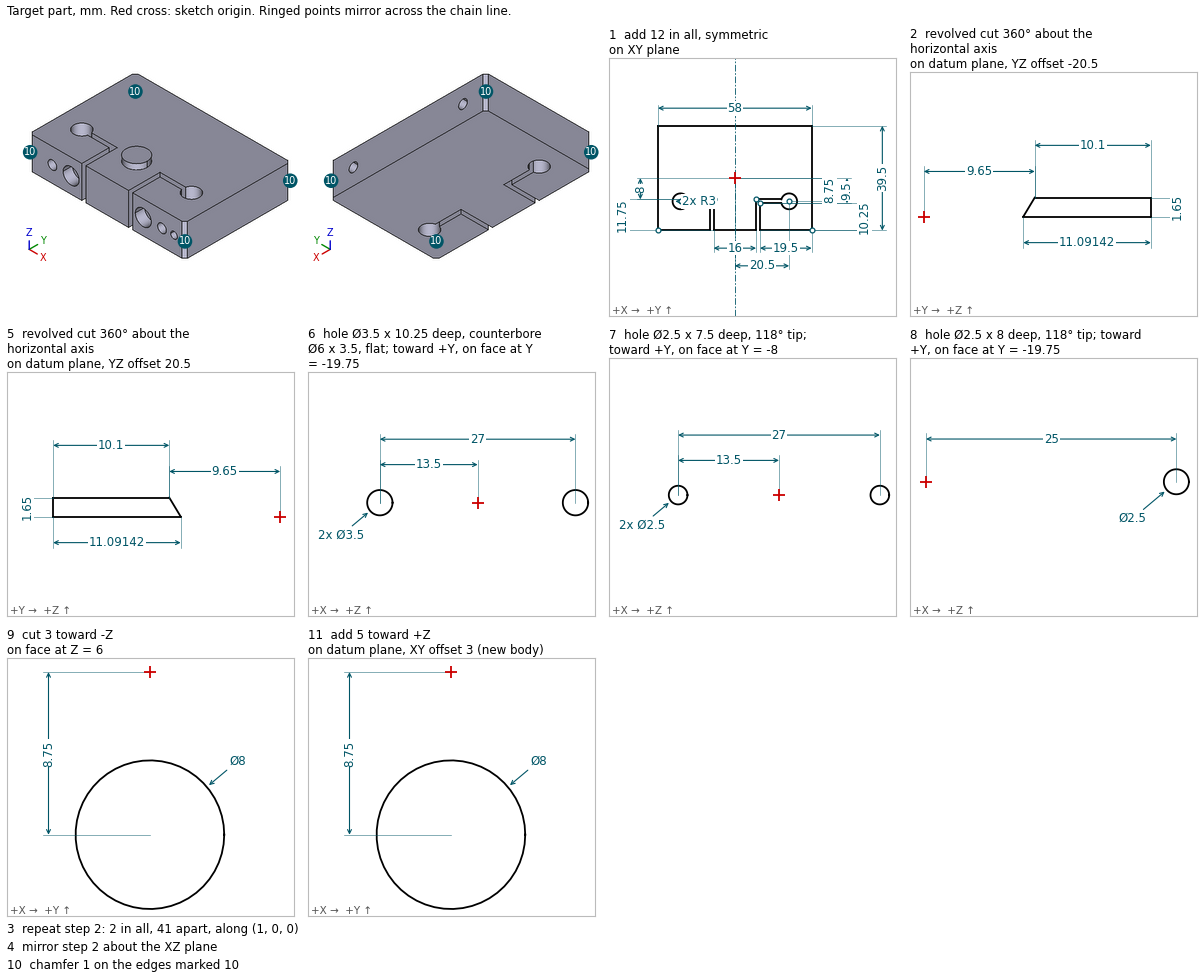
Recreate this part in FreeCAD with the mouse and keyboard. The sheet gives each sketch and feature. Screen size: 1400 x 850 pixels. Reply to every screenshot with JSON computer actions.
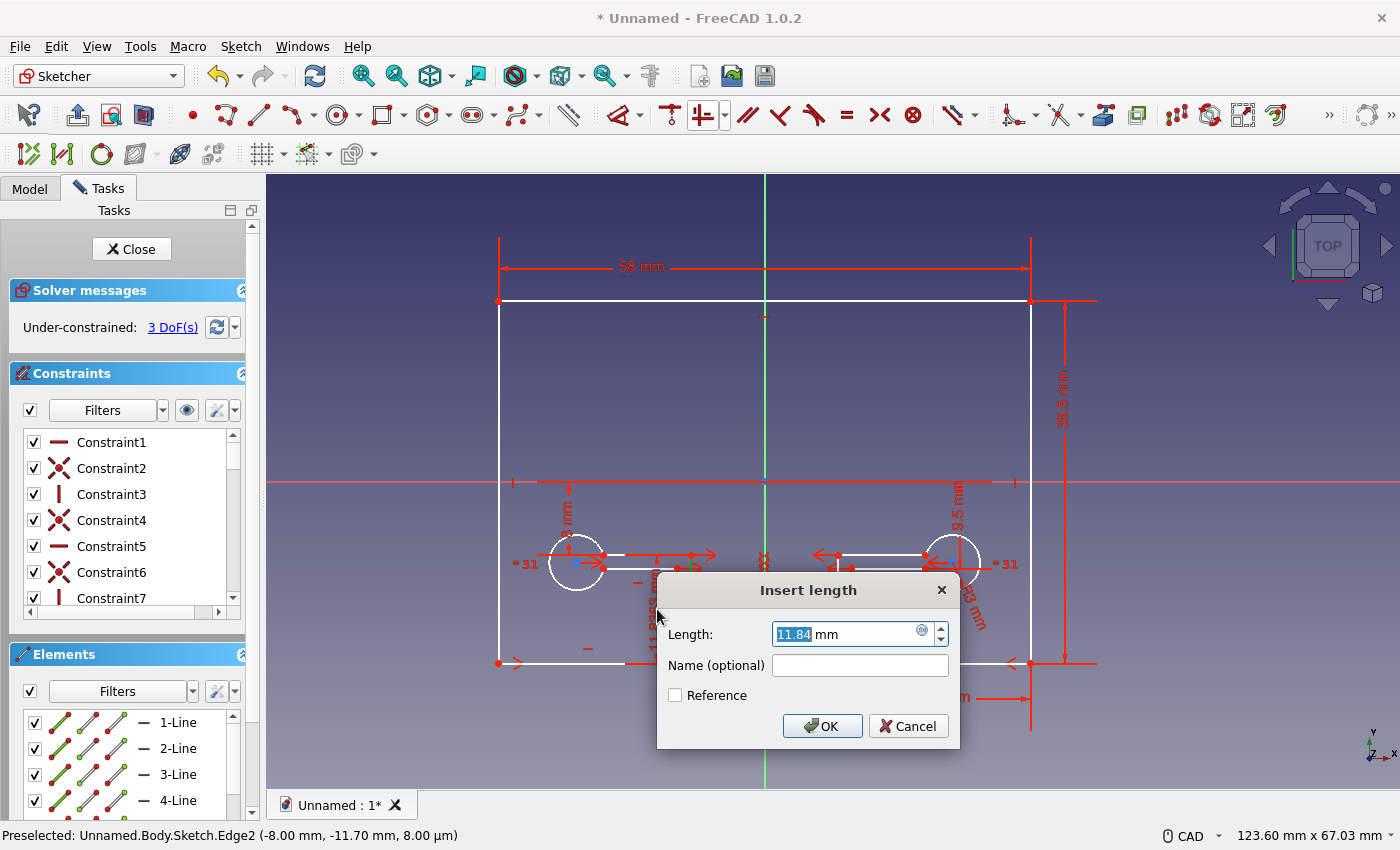
{"action": "type", "text": "11.75"}
{"action": "key", "text": "Return"}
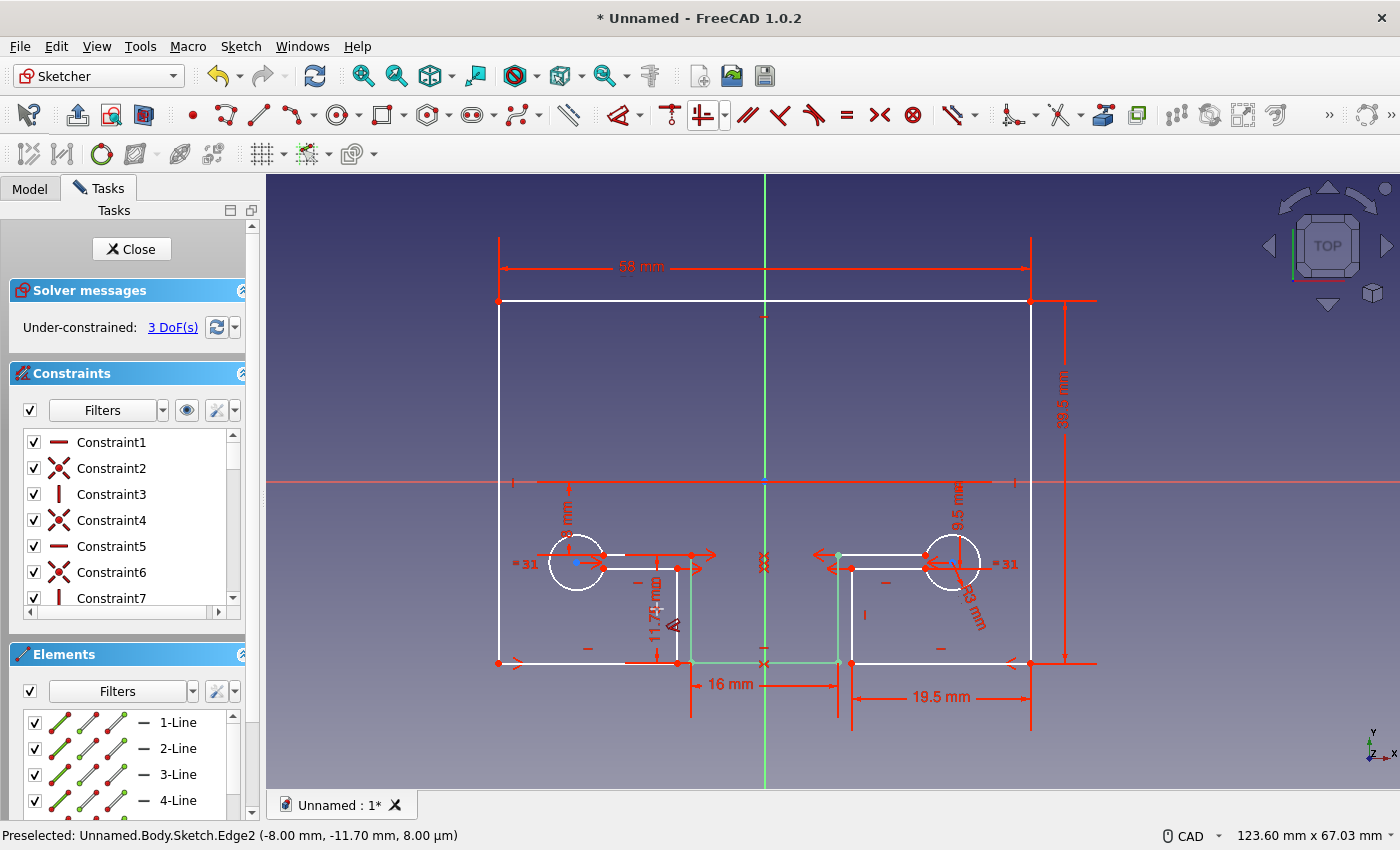
{"action": "left_click", "coordinate": [852, 597]}
{"action": "left_click", "coordinate": [886, 616]}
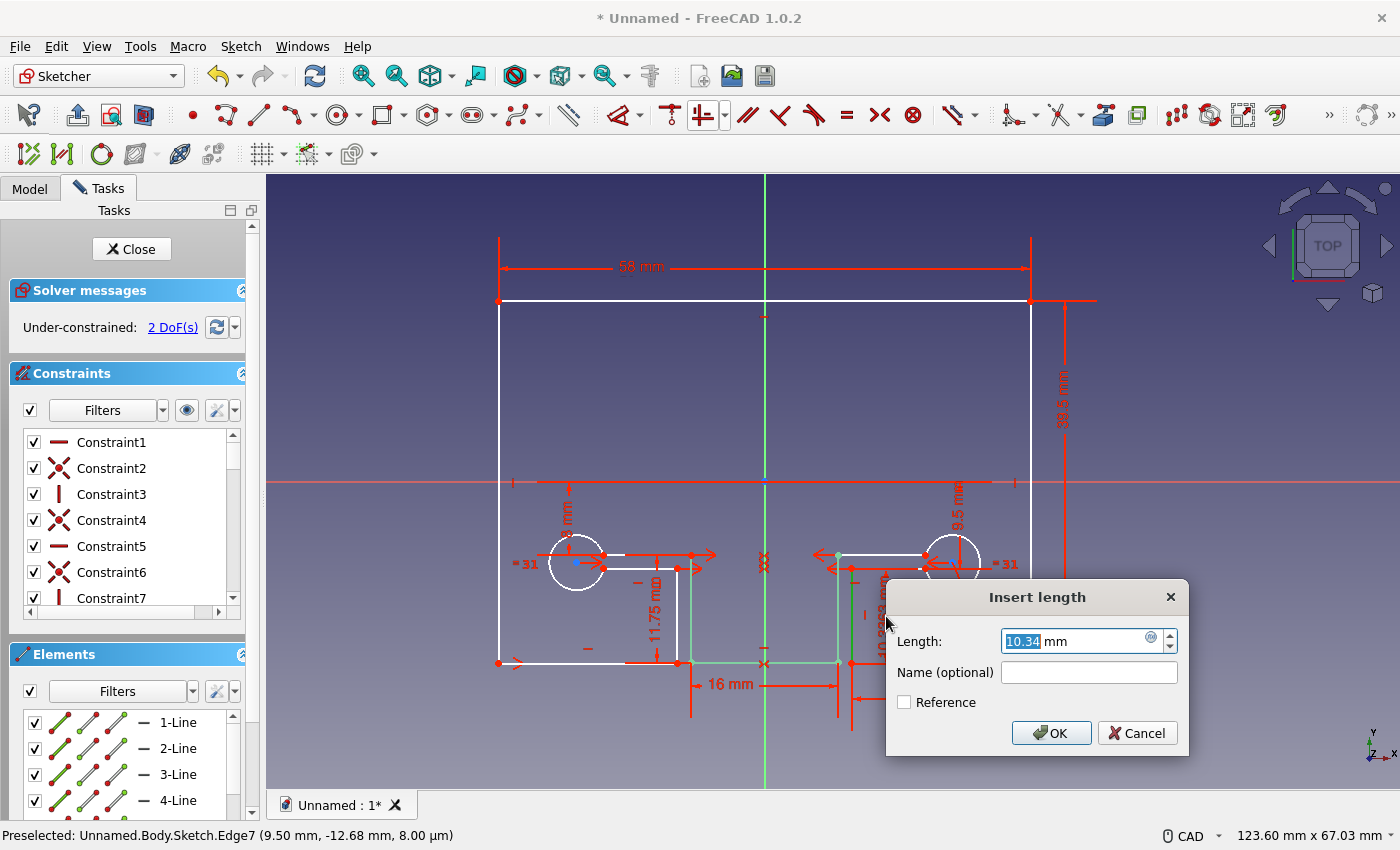
{"action": "type", "text": "10.25"}
{"action": "key", "text": "Return"}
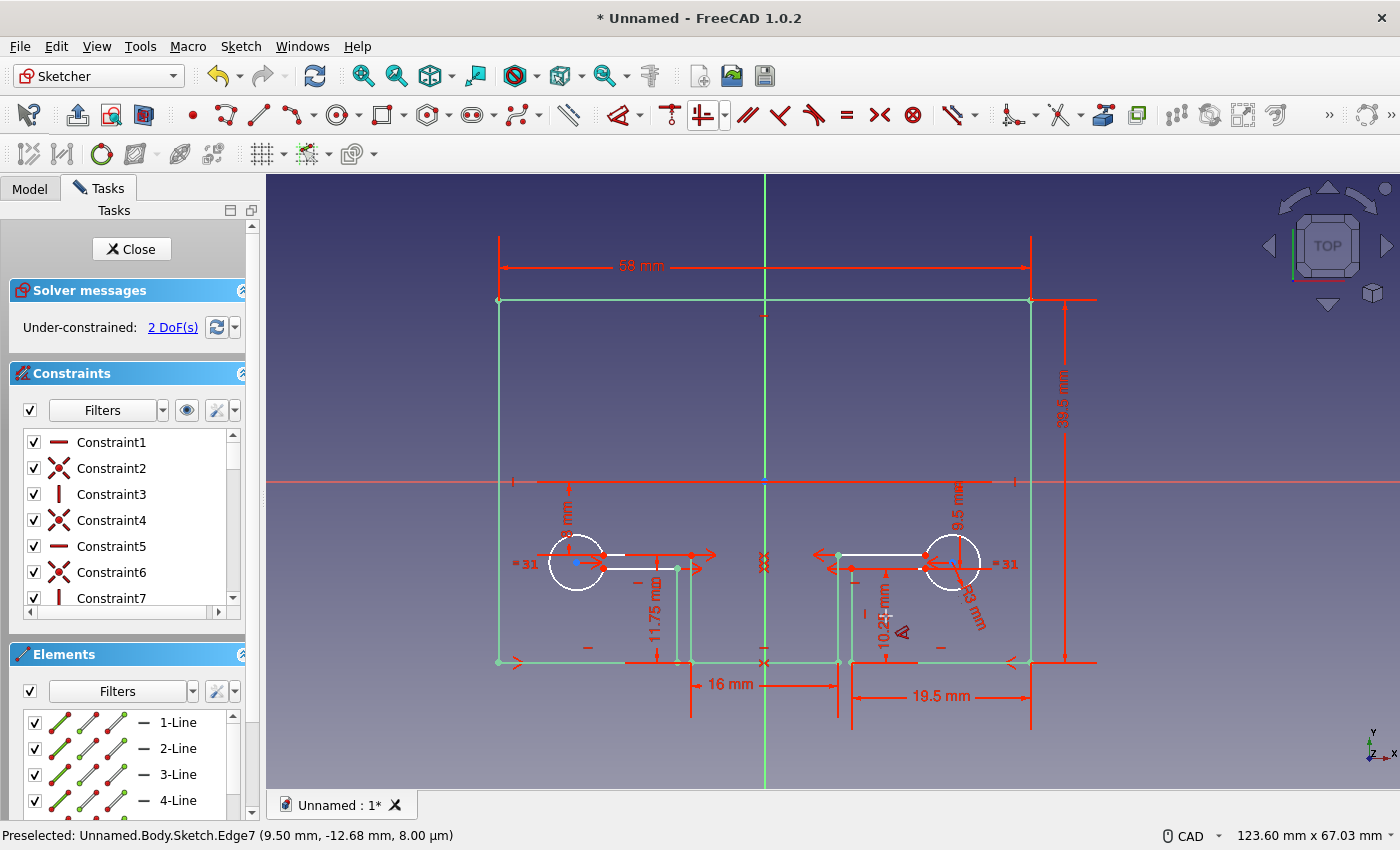
{"action": "left_click", "coordinate": [952, 563]}
{"action": "left_click", "coordinate": [815, 597]}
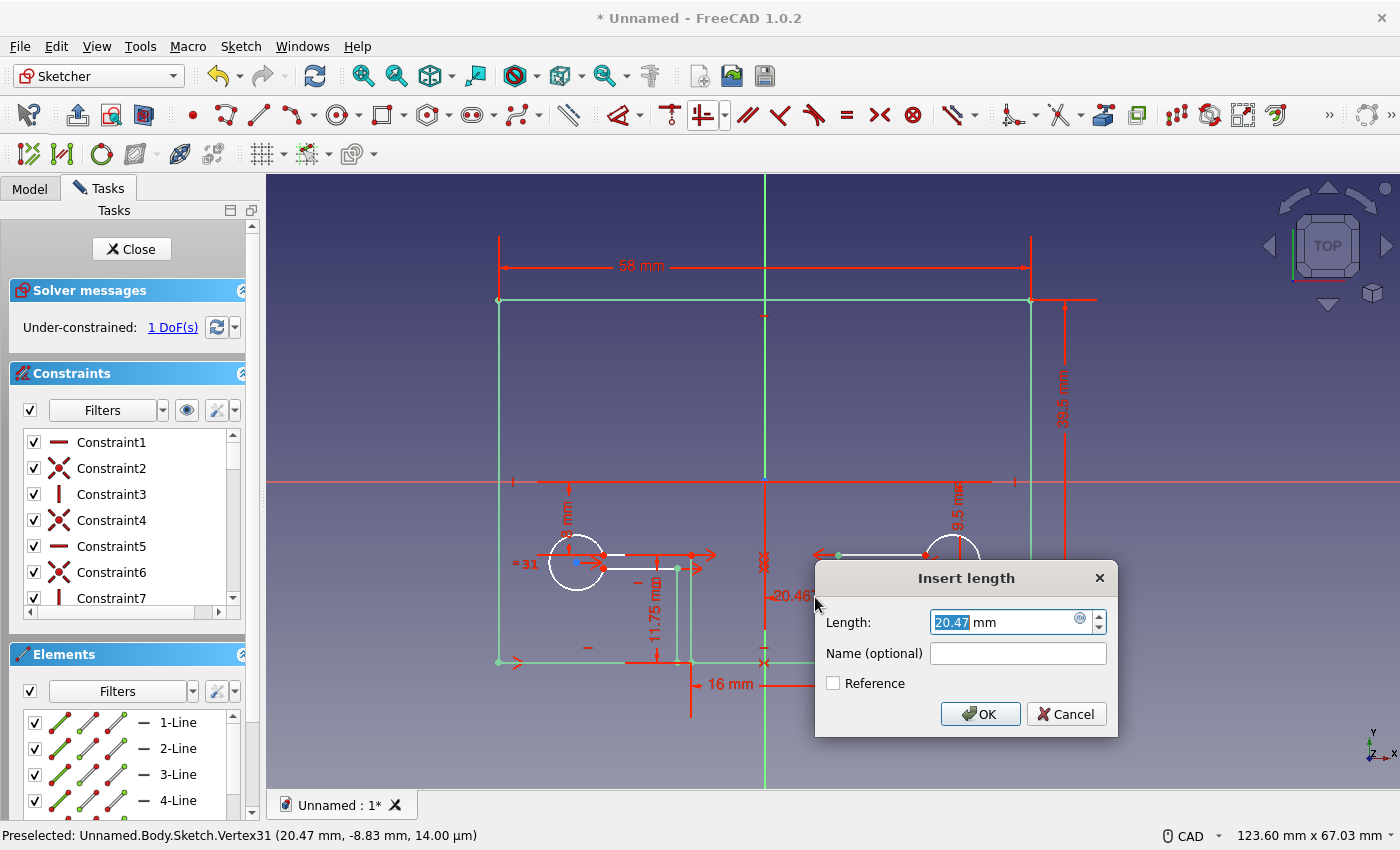
{"action": "type", "text": "20.5"}
{"action": "key", "text": "Return"}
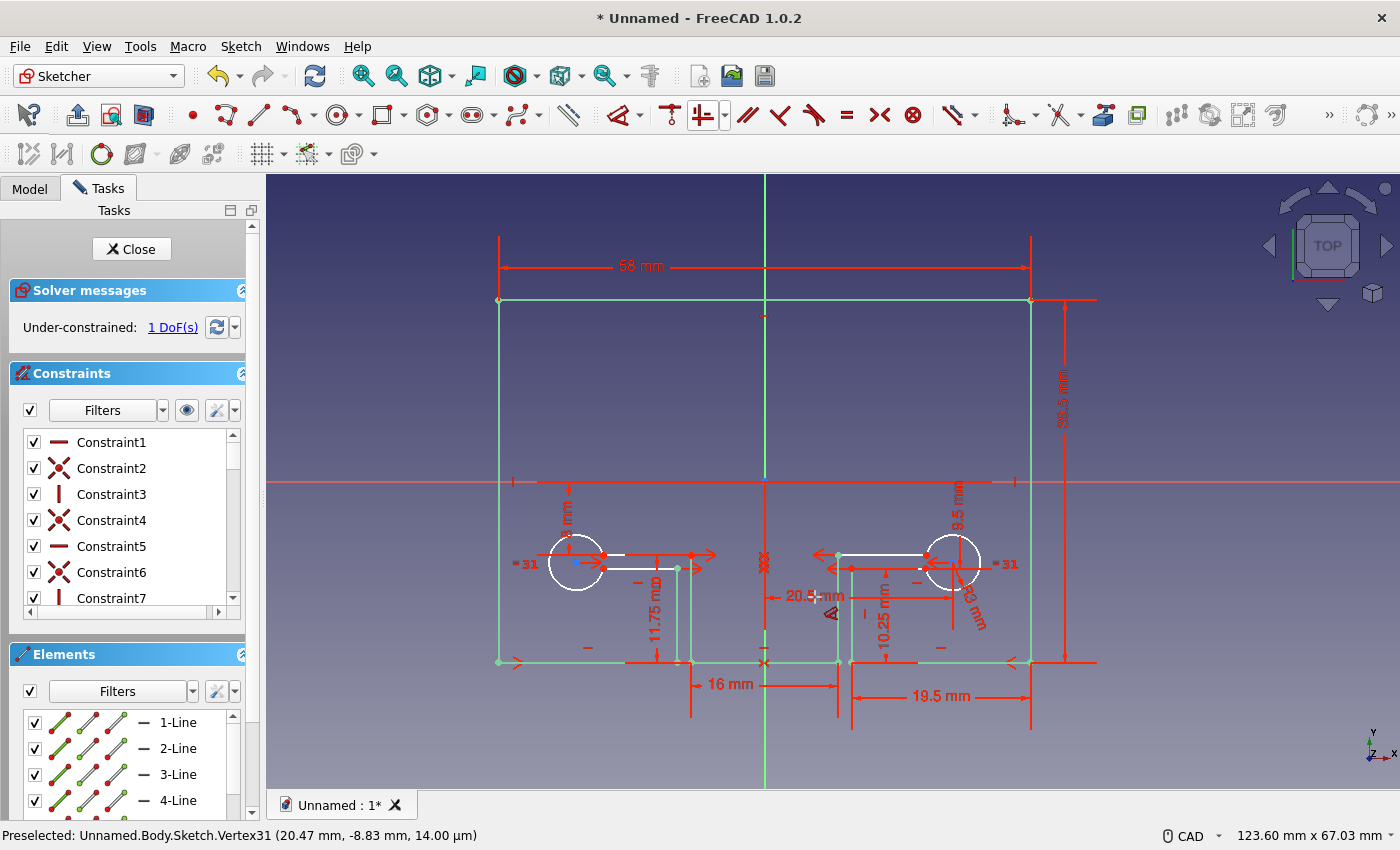
{"action": "left_click", "coordinate": [953, 563]}
{"action": "left_click", "coordinate": [731, 522]}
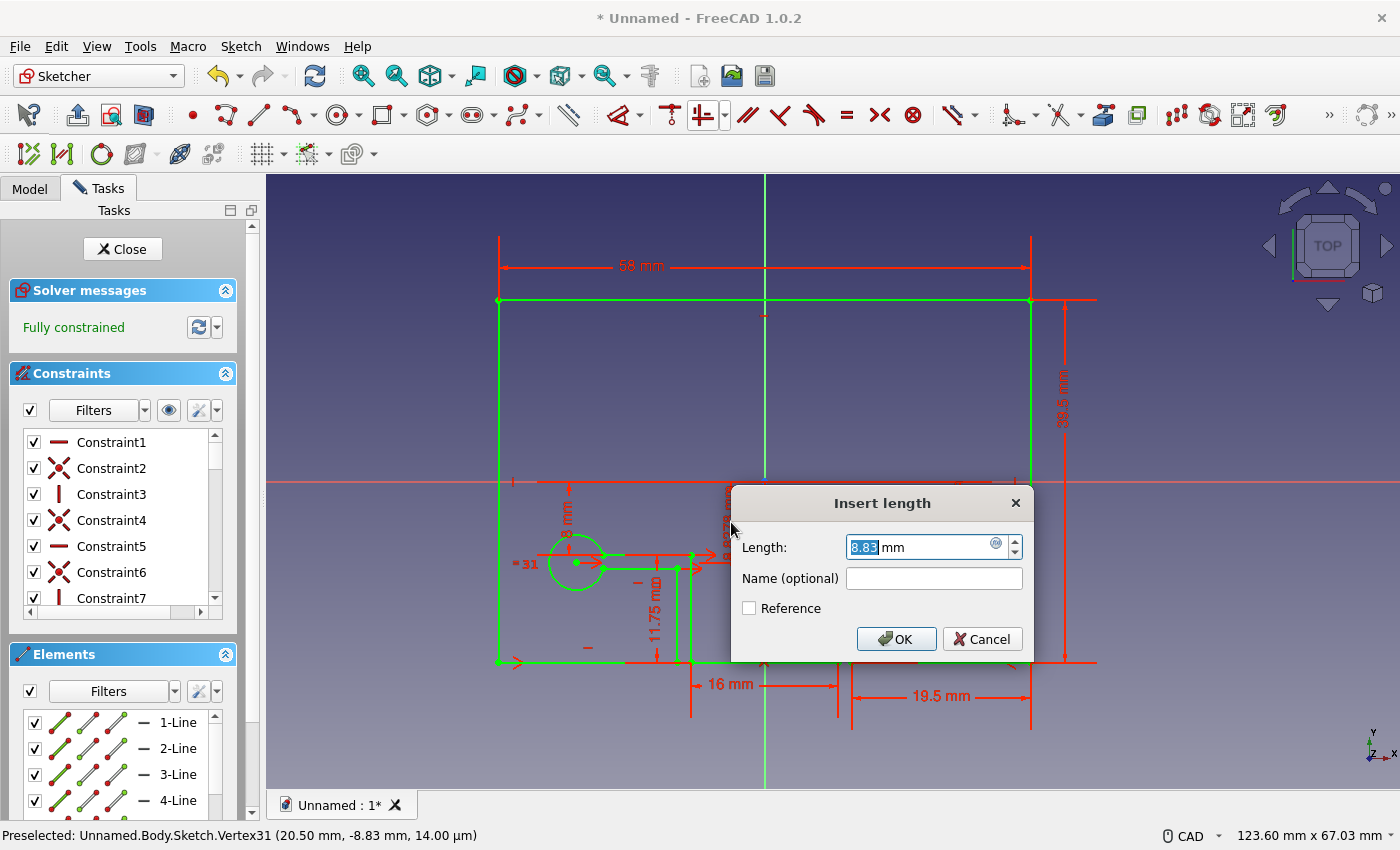
{"action": "type", "text": "8.75"}
{"action": "key", "text": "Return"}
{"action": "key", "text": "Escape"}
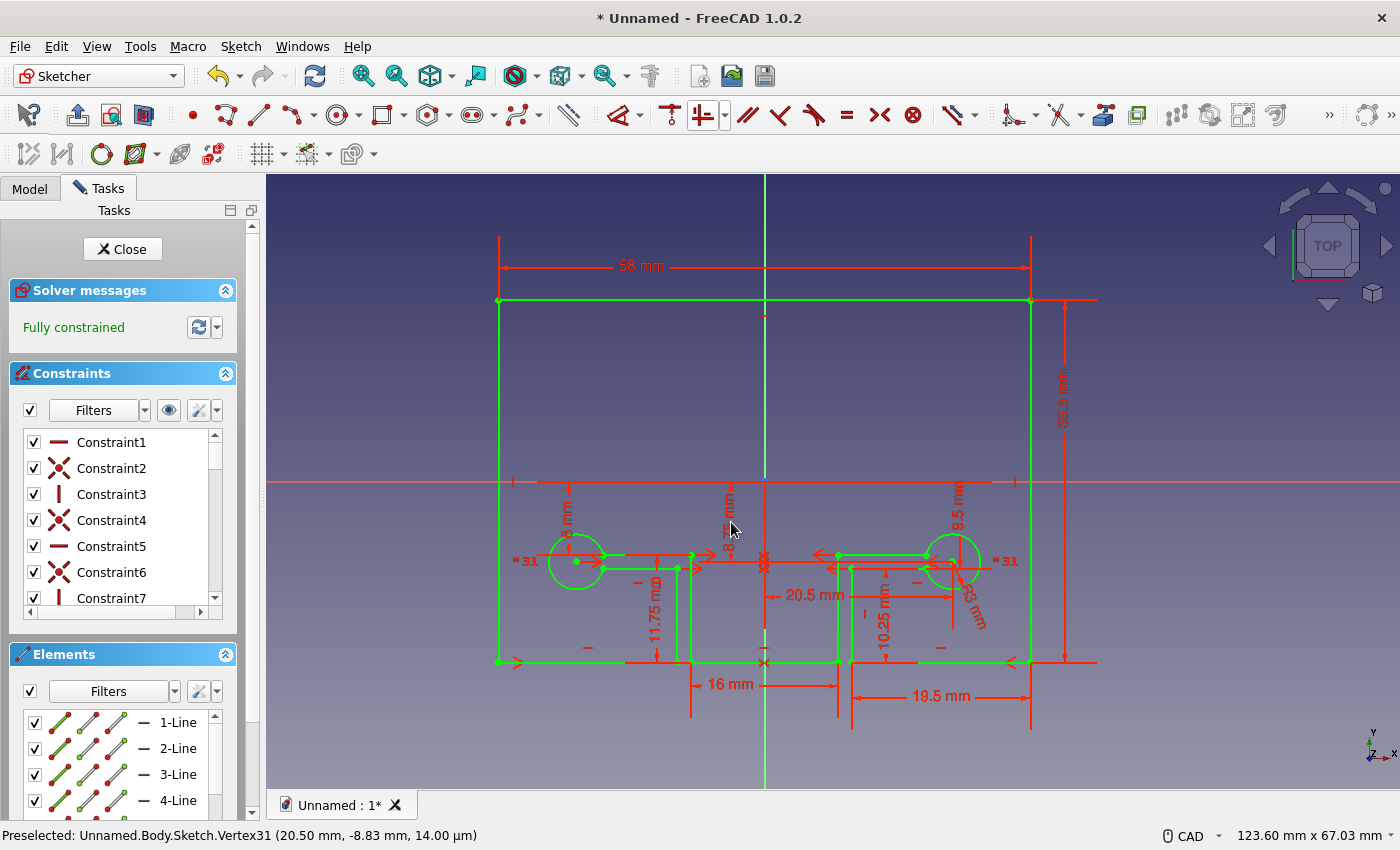
{"action": "left_click", "coordinate": [123, 249]}